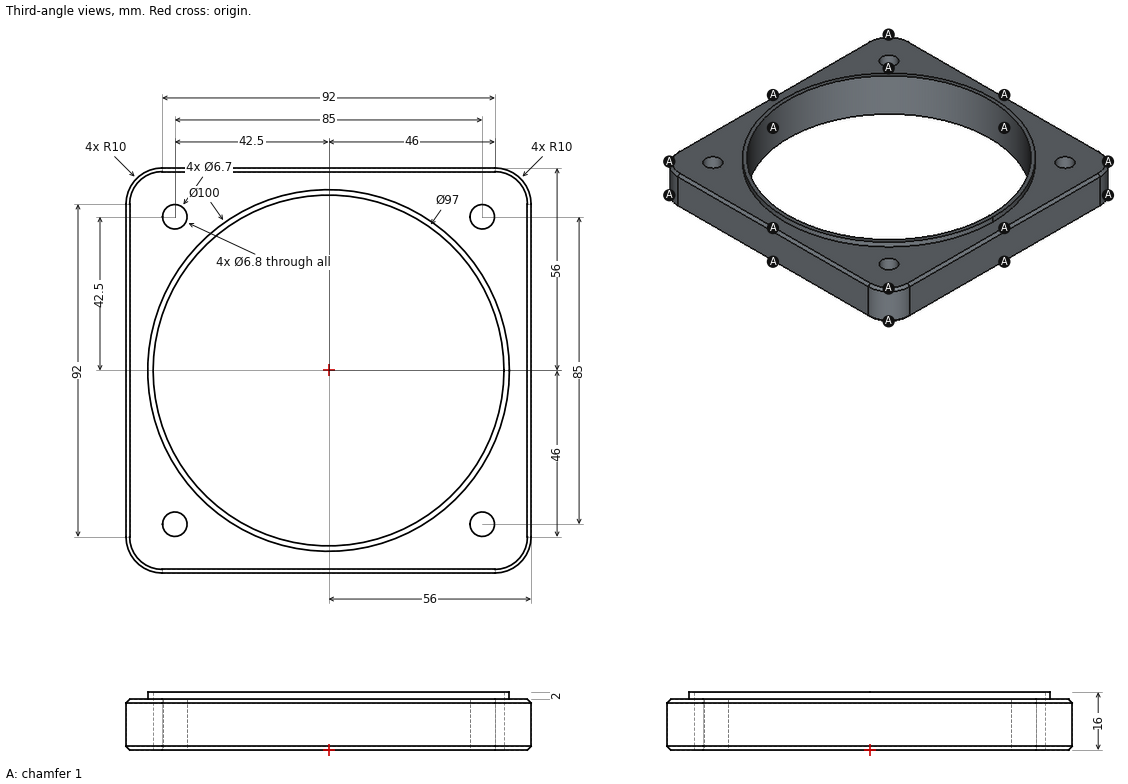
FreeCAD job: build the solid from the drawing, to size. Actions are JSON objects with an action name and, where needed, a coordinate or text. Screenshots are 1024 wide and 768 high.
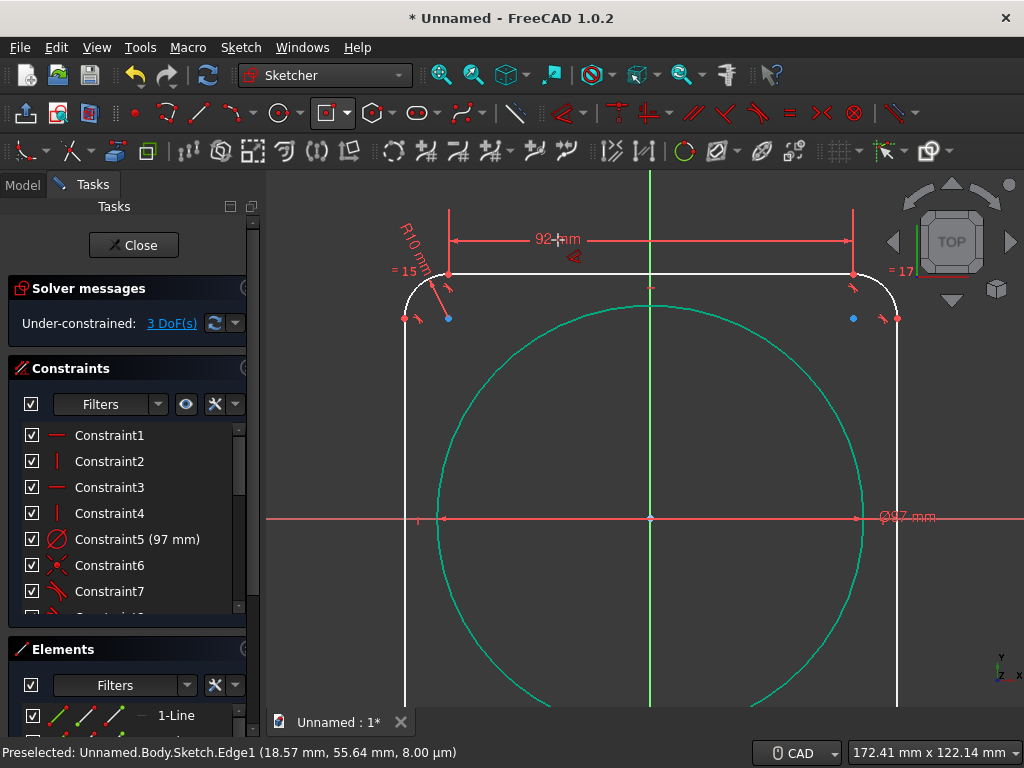
{"action": "left_click", "coordinate": [405, 440]}
{"action": "left_click", "coordinate": [371, 499]}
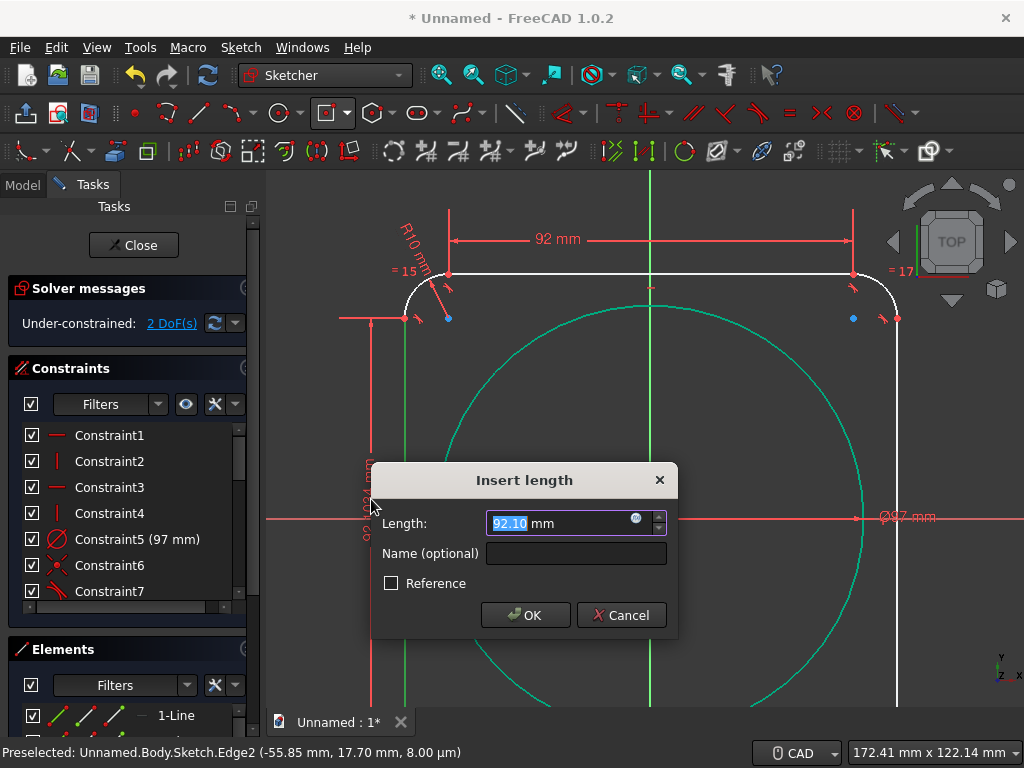
{"action": "type", "text": "92"}
{"action": "key", "text": "Return"}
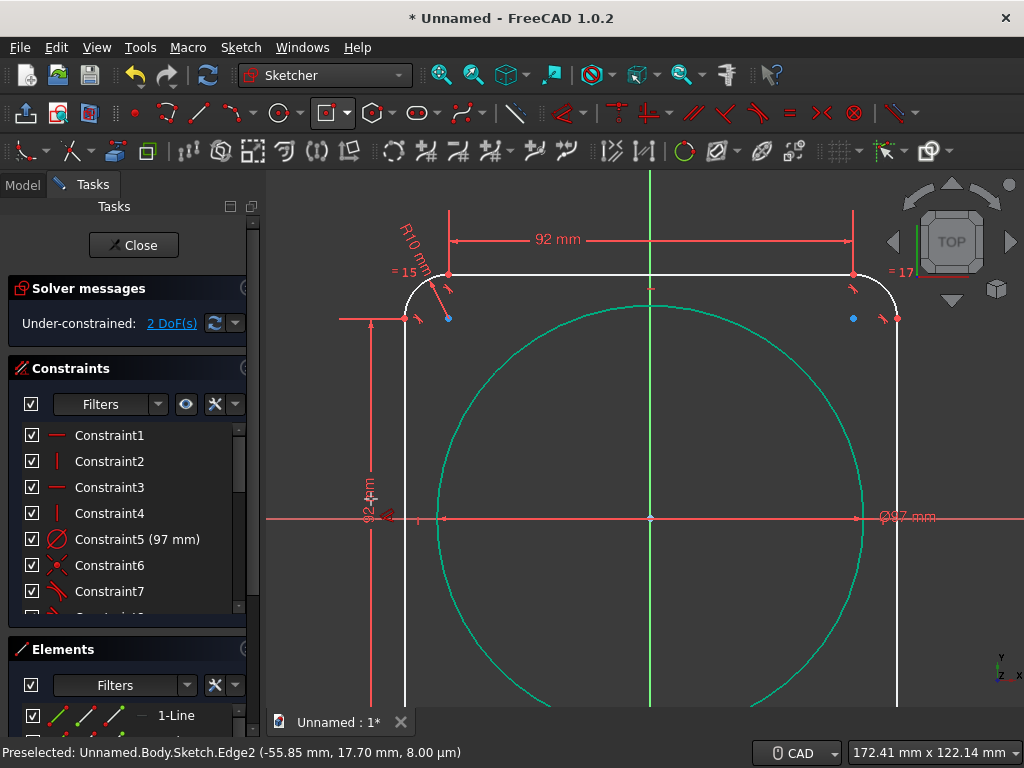
{"action": "left_click", "coordinate": [853, 275]}
{"action": "left_click", "coordinate": [752, 241]}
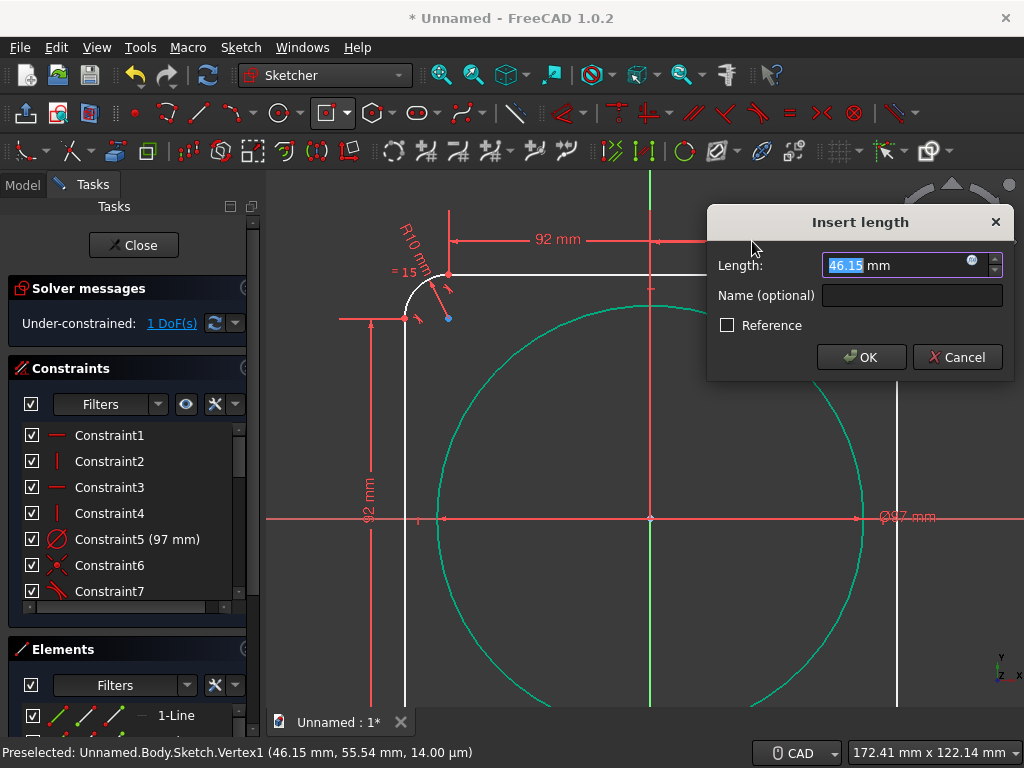
{"action": "type", "text": "46"}
{"action": "key", "text": "Return"}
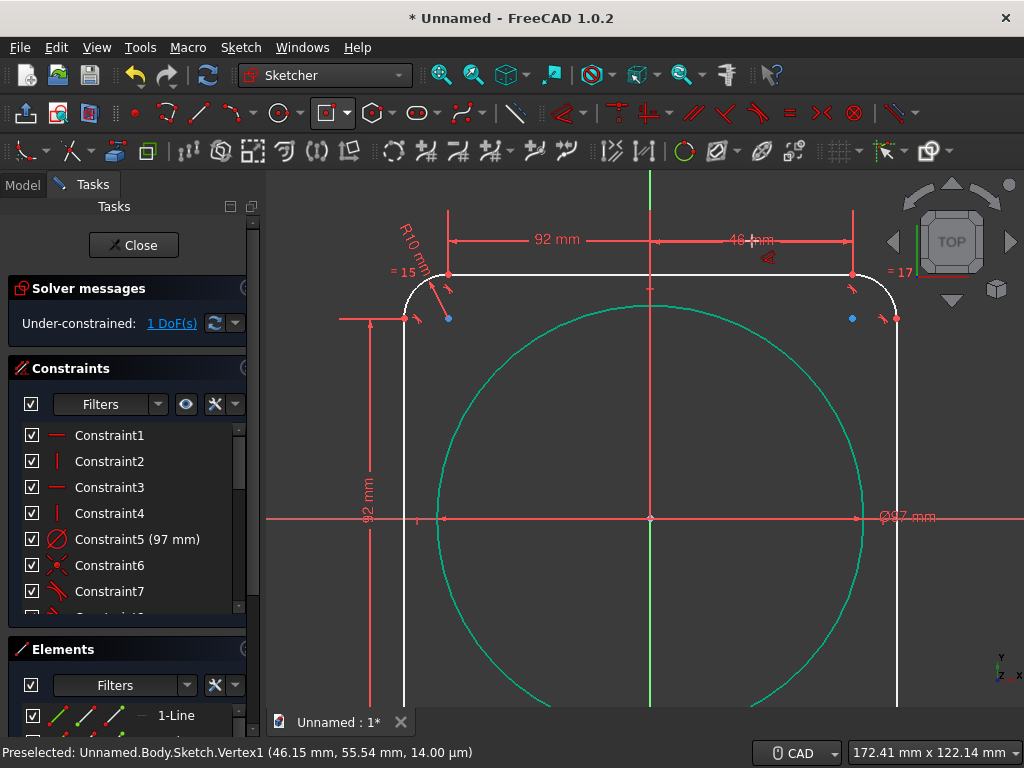
{"action": "left_click", "coordinate": [853, 275]}
{"action": "left_click", "coordinate": [616, 397]}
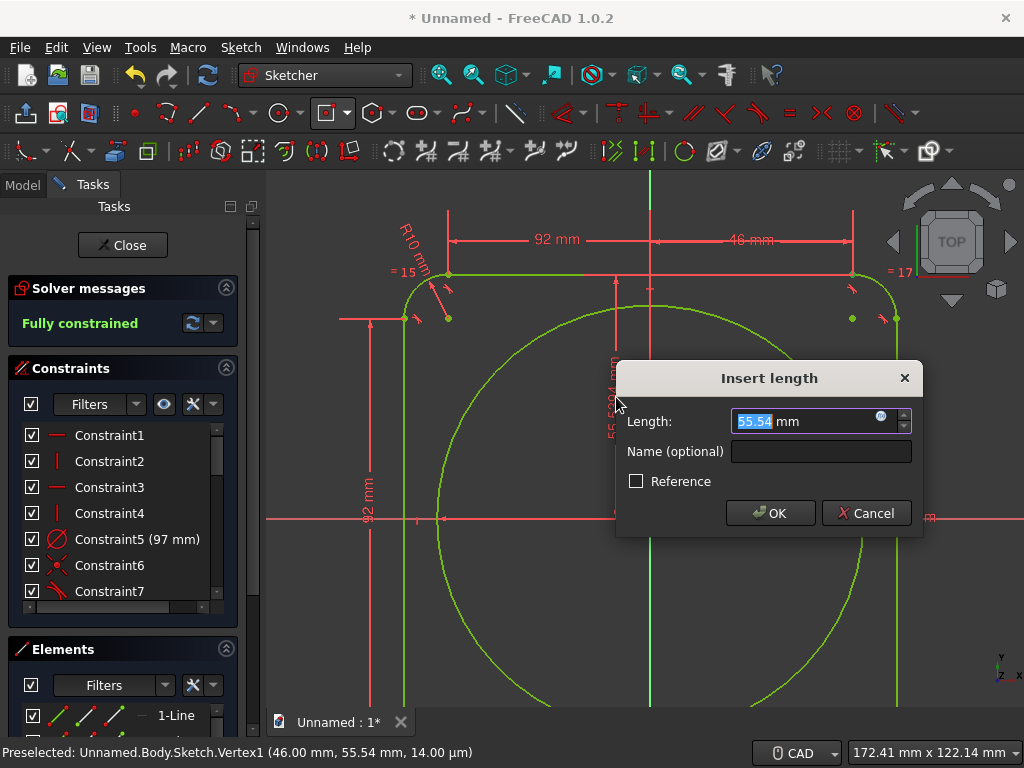
{"action": "type", "text": "56"}
{"action": "key", "text": "Return"}
{"action": "key", "text": "Escape"}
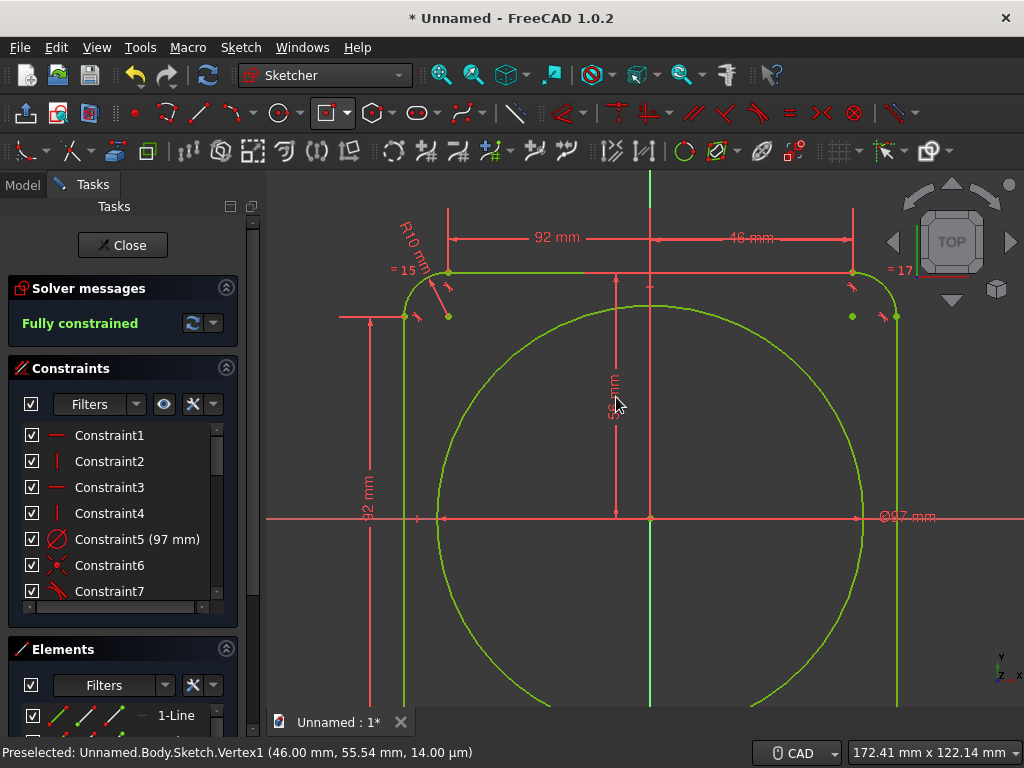
{"action": "left_click", "coordinate": [123, 245]}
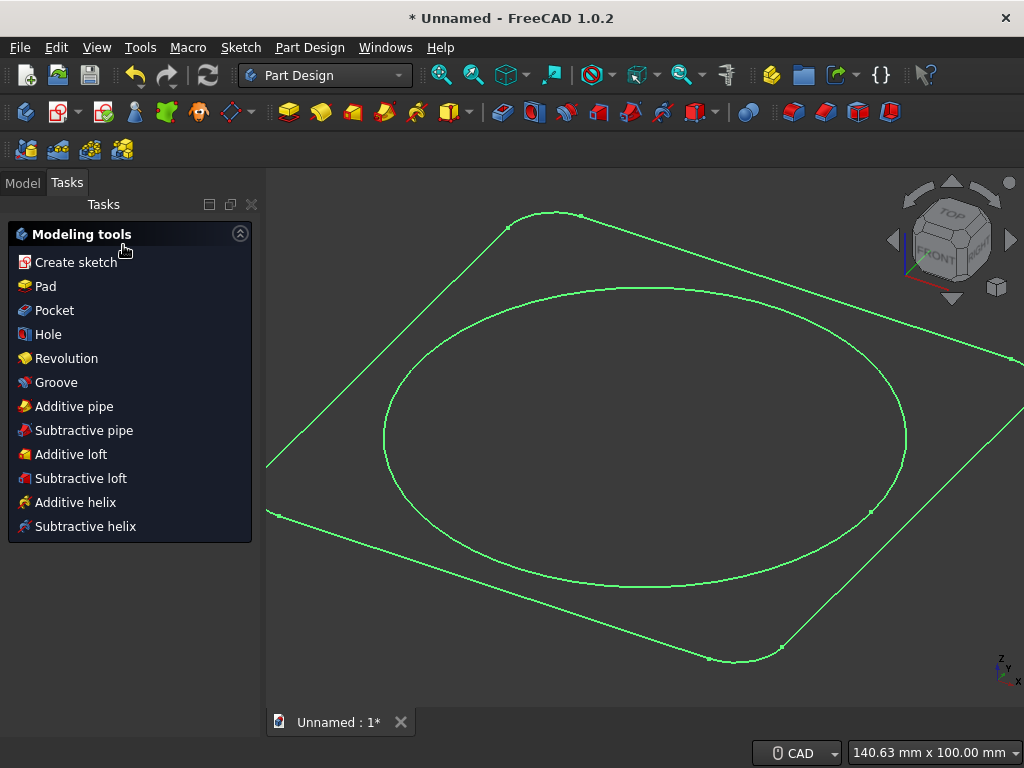
{"action": "left_click", "coordinate": [290, 112]}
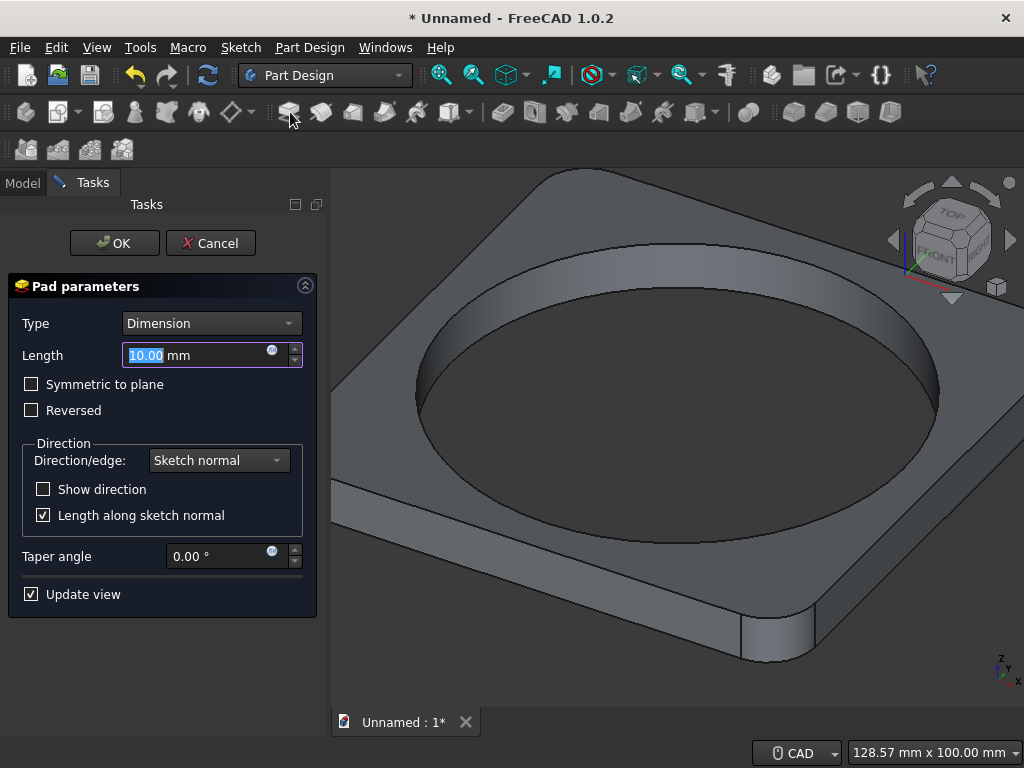
{"action": "type", "text": "16"}
{"action": "key", "text": "Tab"}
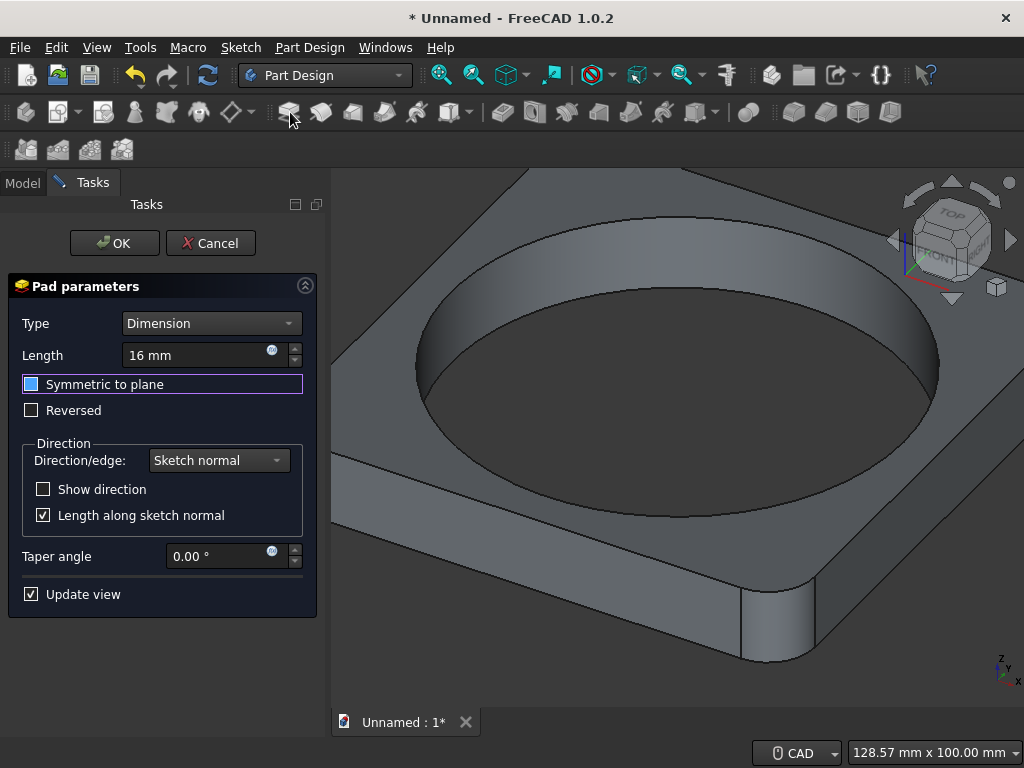
{"action": "left_click", "coordinate": [115, 243]}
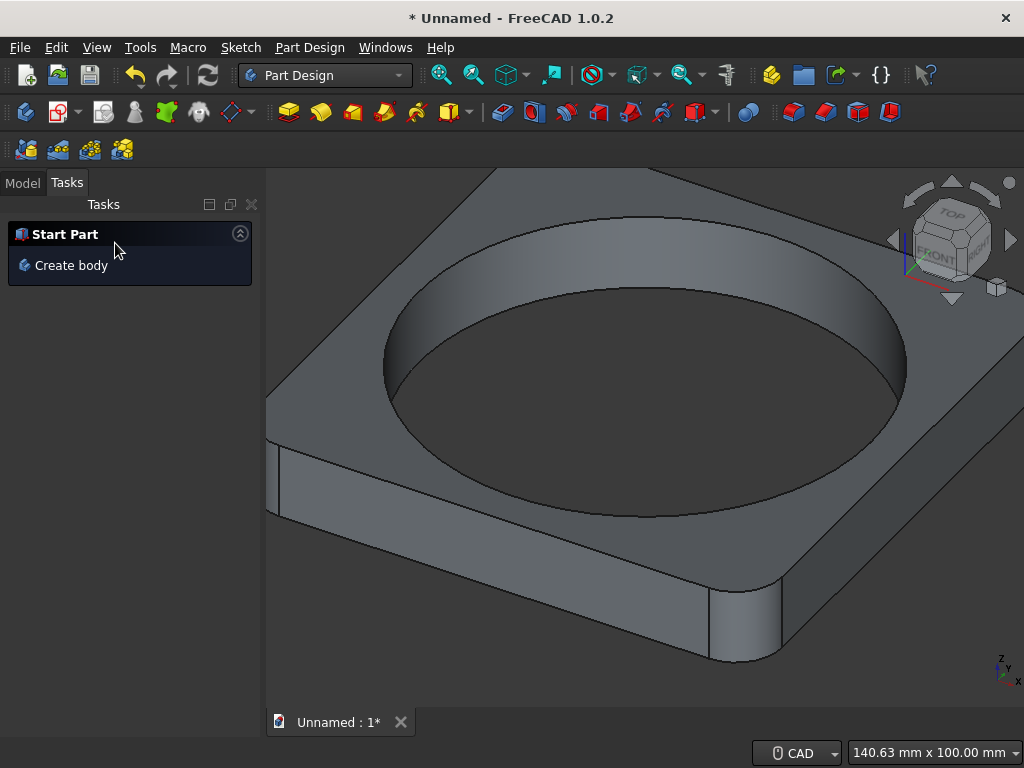
{"action": "left_click", "coordinate": [442, 76]}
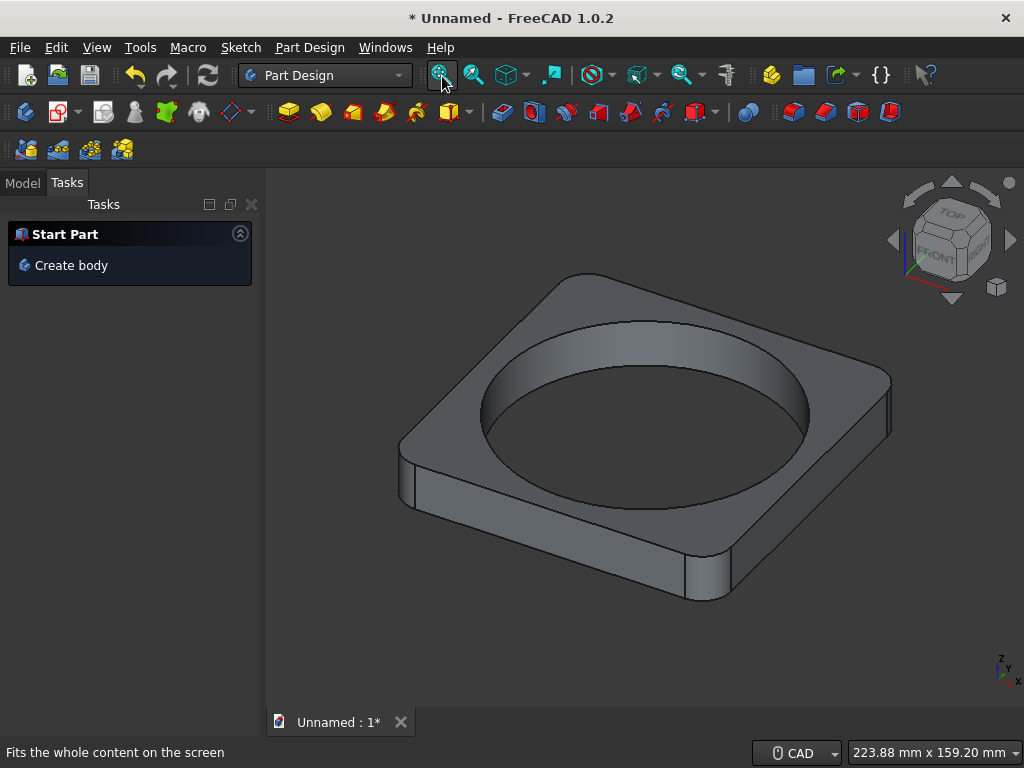
{"action": "left_click", "coordinate": [558, 314]}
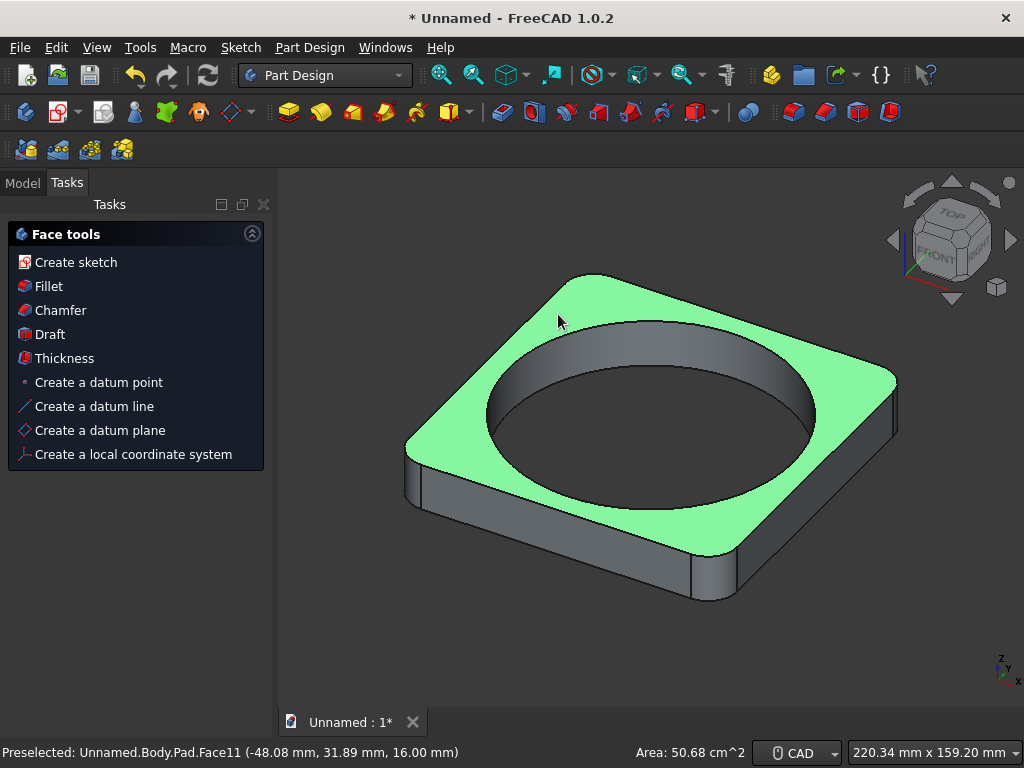
{"action": "left_click", "coordinate": [58, 112]}